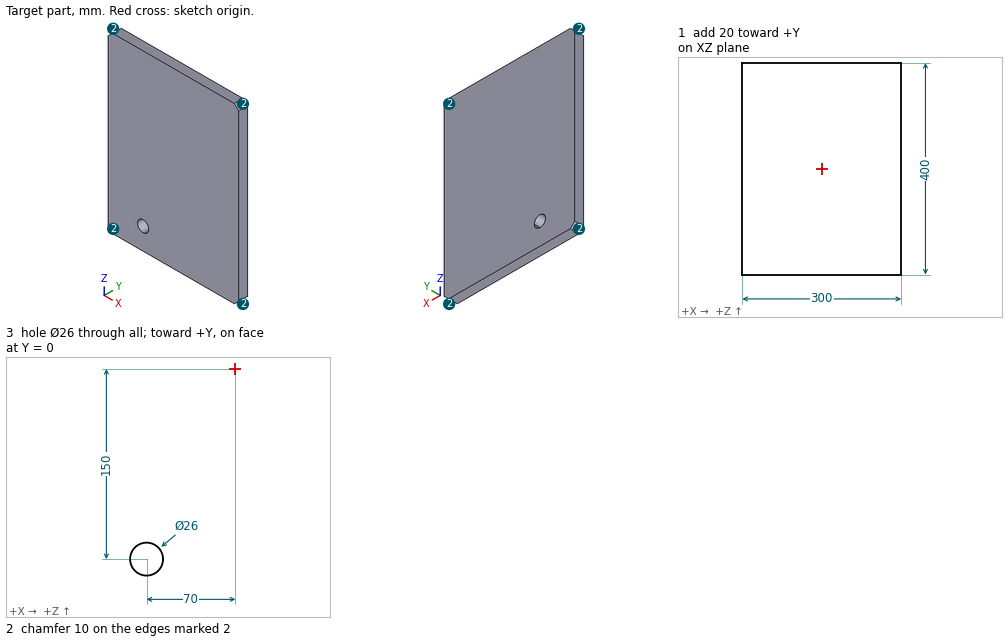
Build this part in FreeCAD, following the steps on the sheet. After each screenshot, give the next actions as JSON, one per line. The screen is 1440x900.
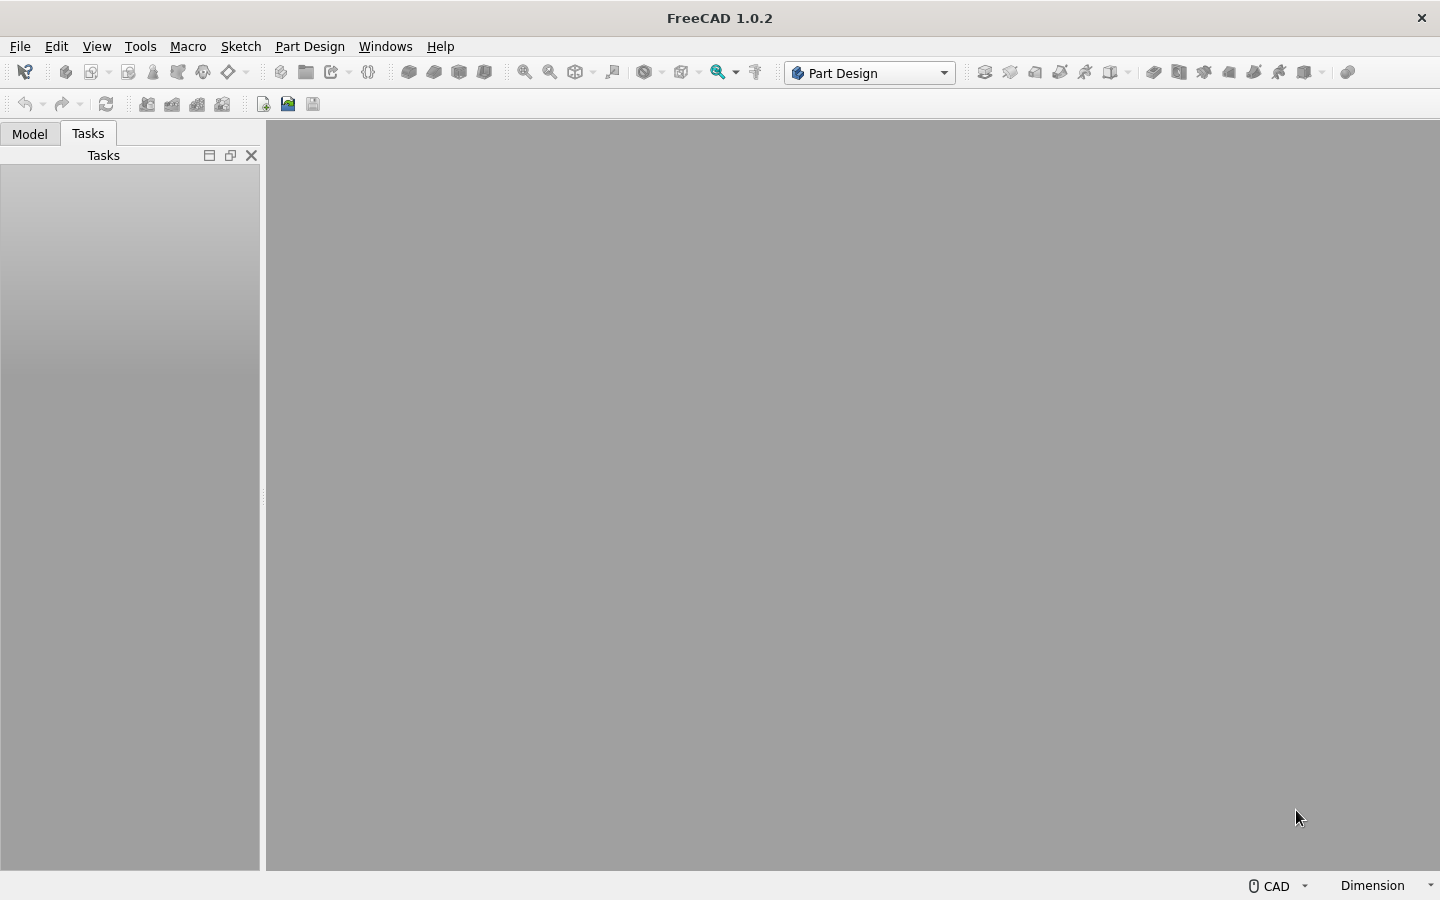
{"action": "left_click", "coordinate": [263, 104]}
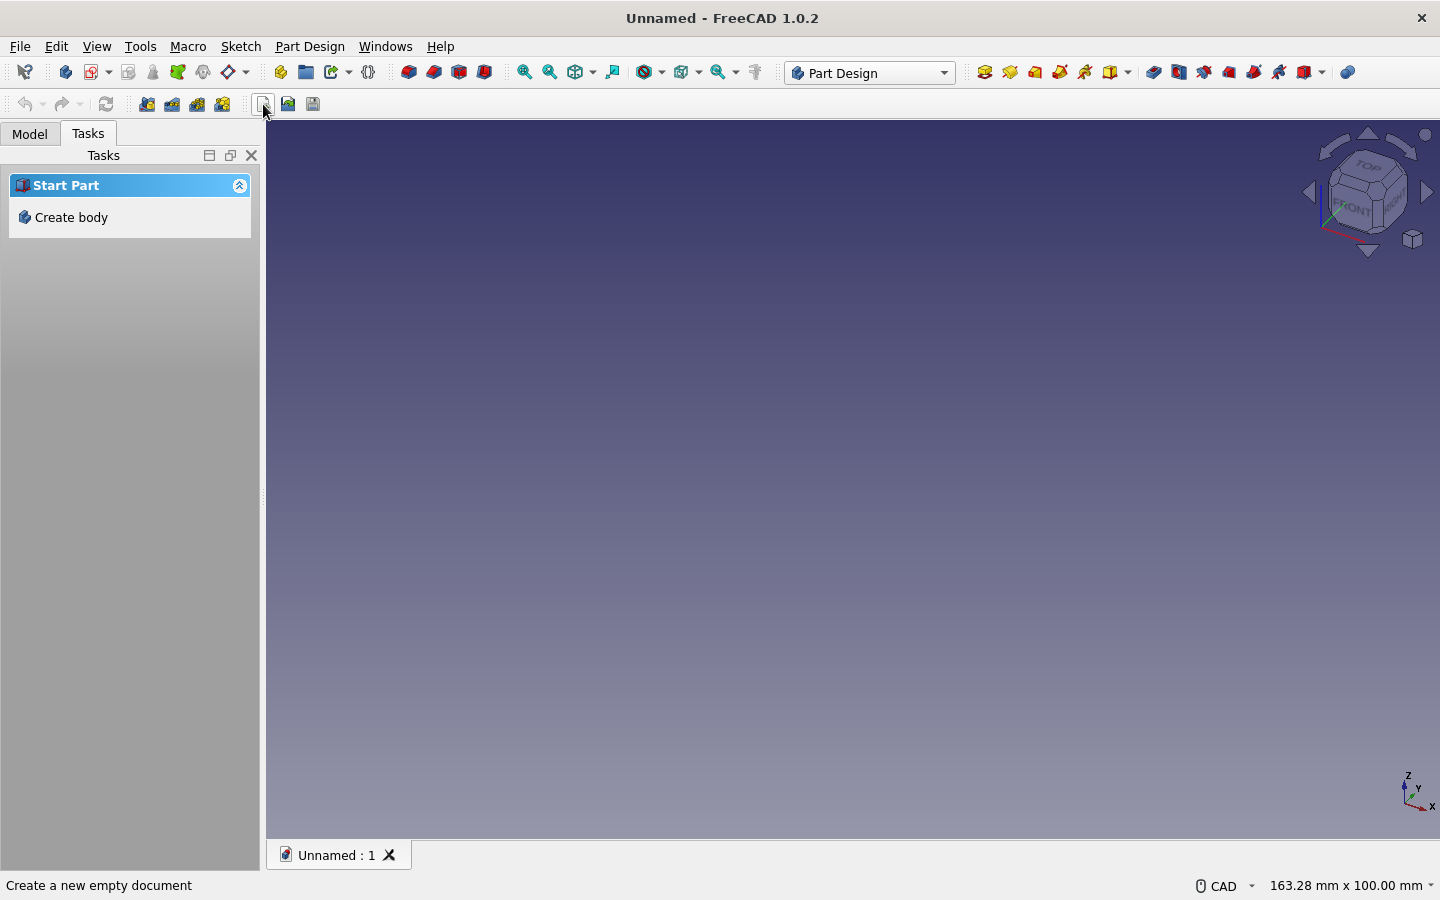
{"action": "left_click", "coordinate": [90, 72]}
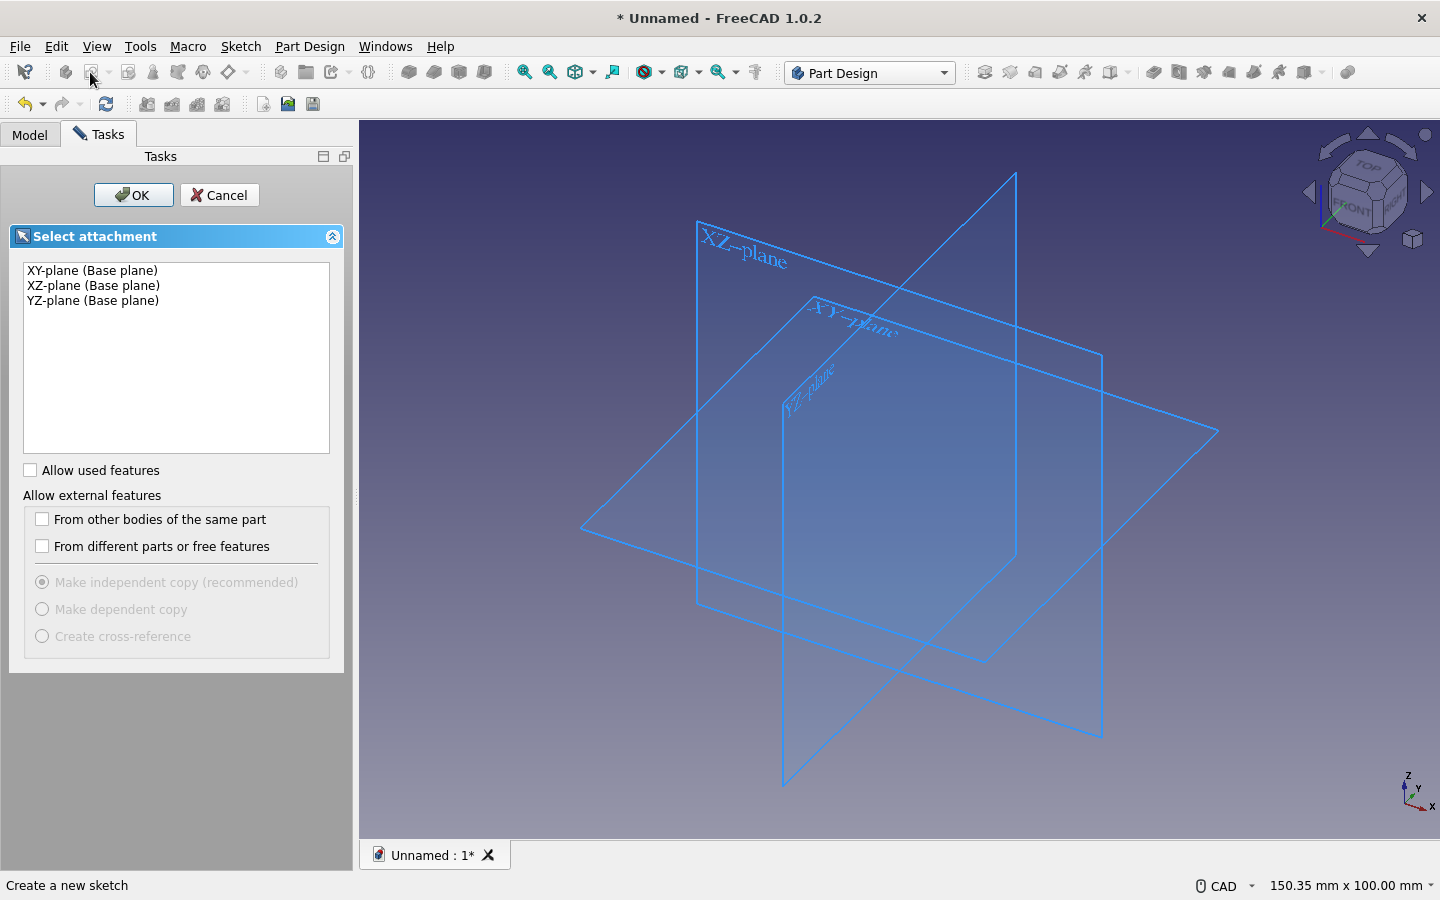
{"action": "left_click", "coordinate": [84, 286]}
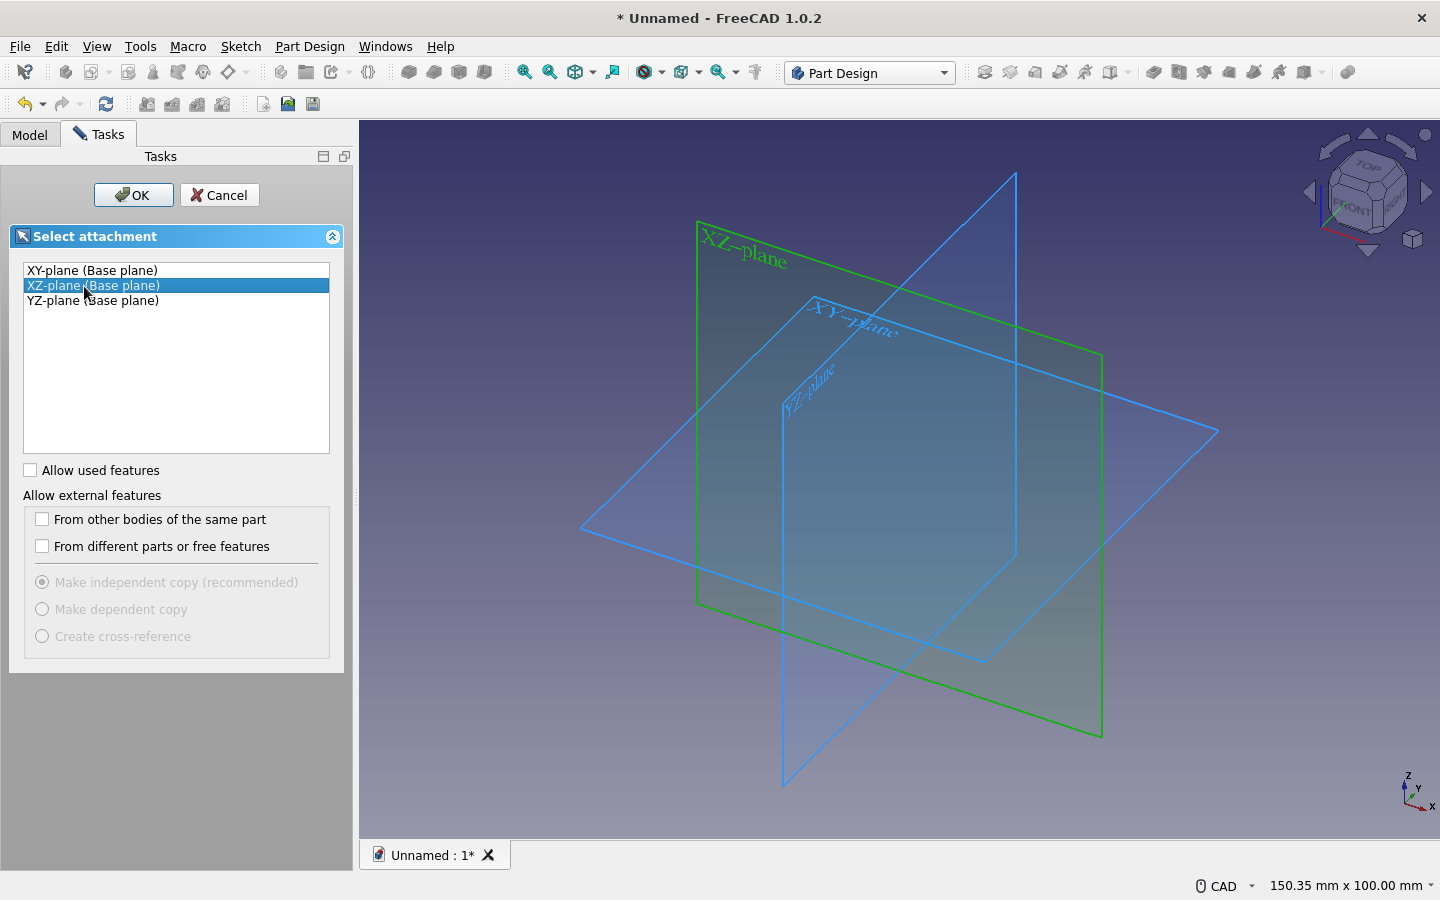
{"action": "left_click", "coordinate": [134, 195]}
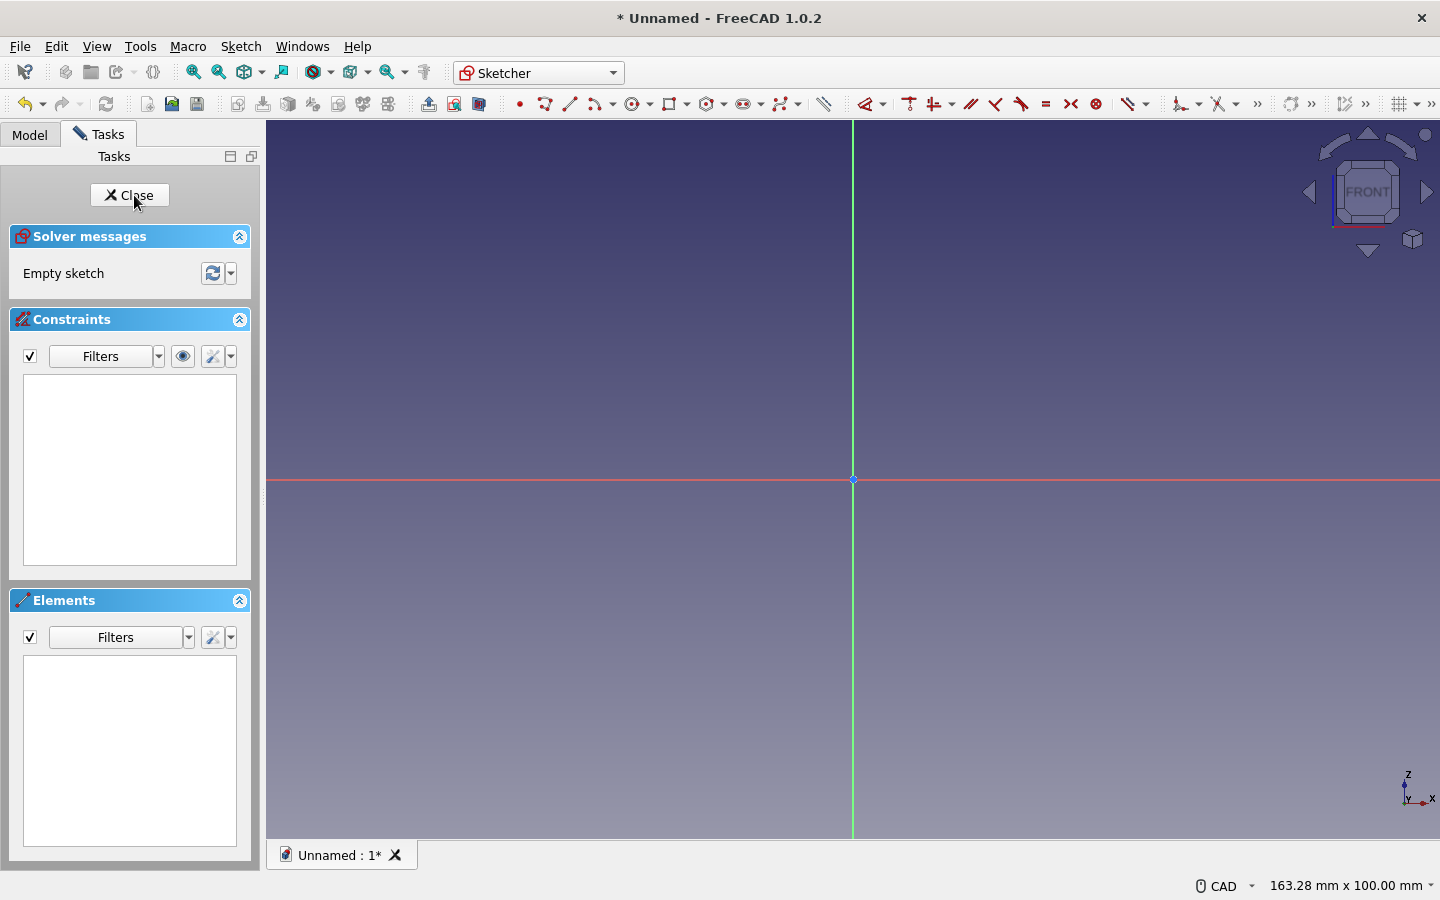
{"action": "scroll", "coordinate": [771, 480], "scroll_direction": "down", "scroll_amount": 9}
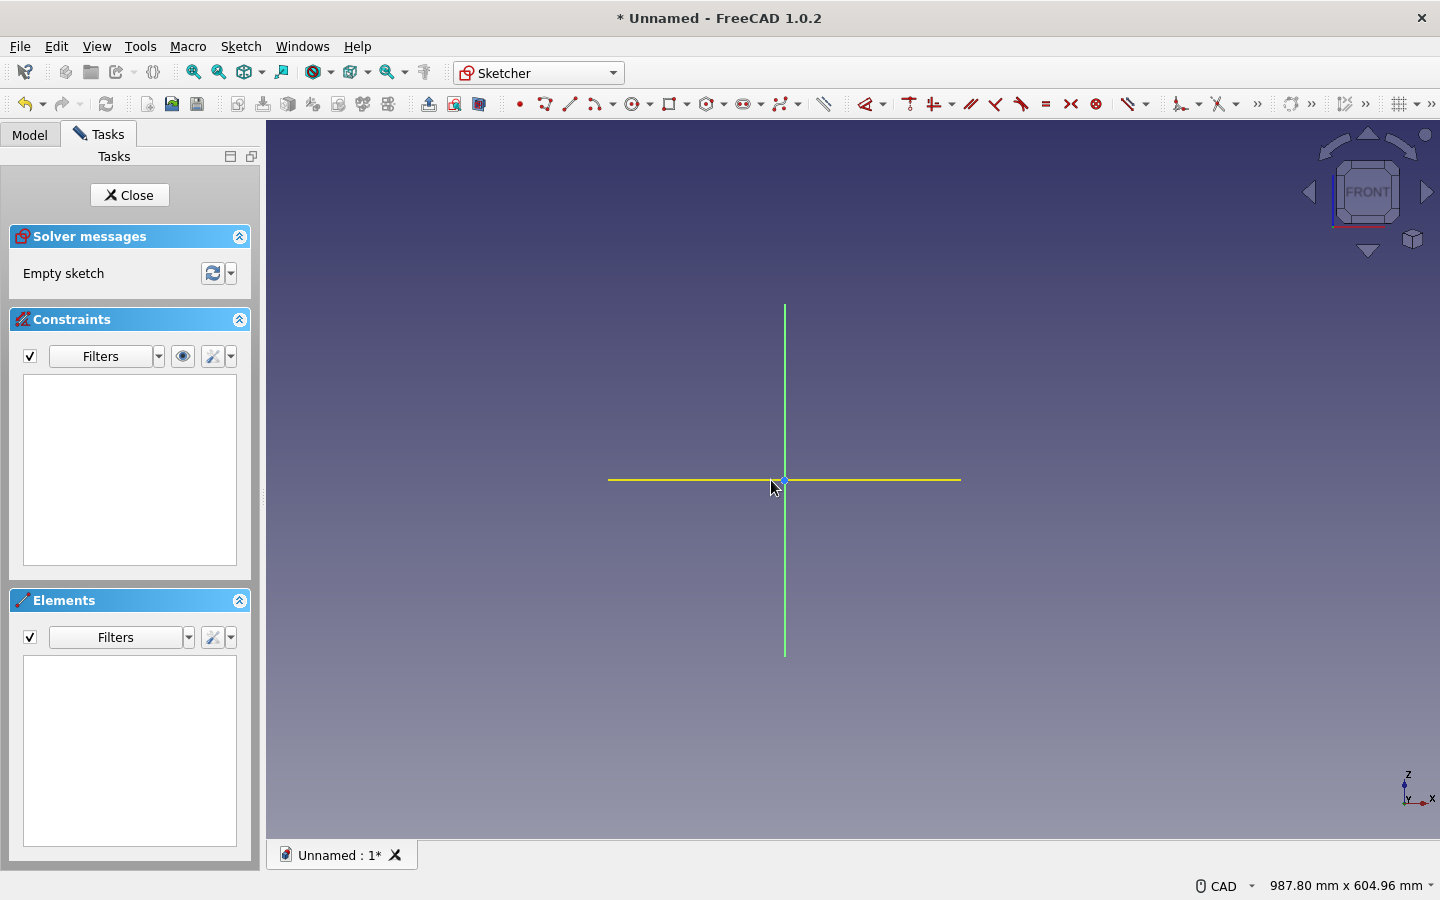
{"action": "left_click", "coordinate": [686, 104]}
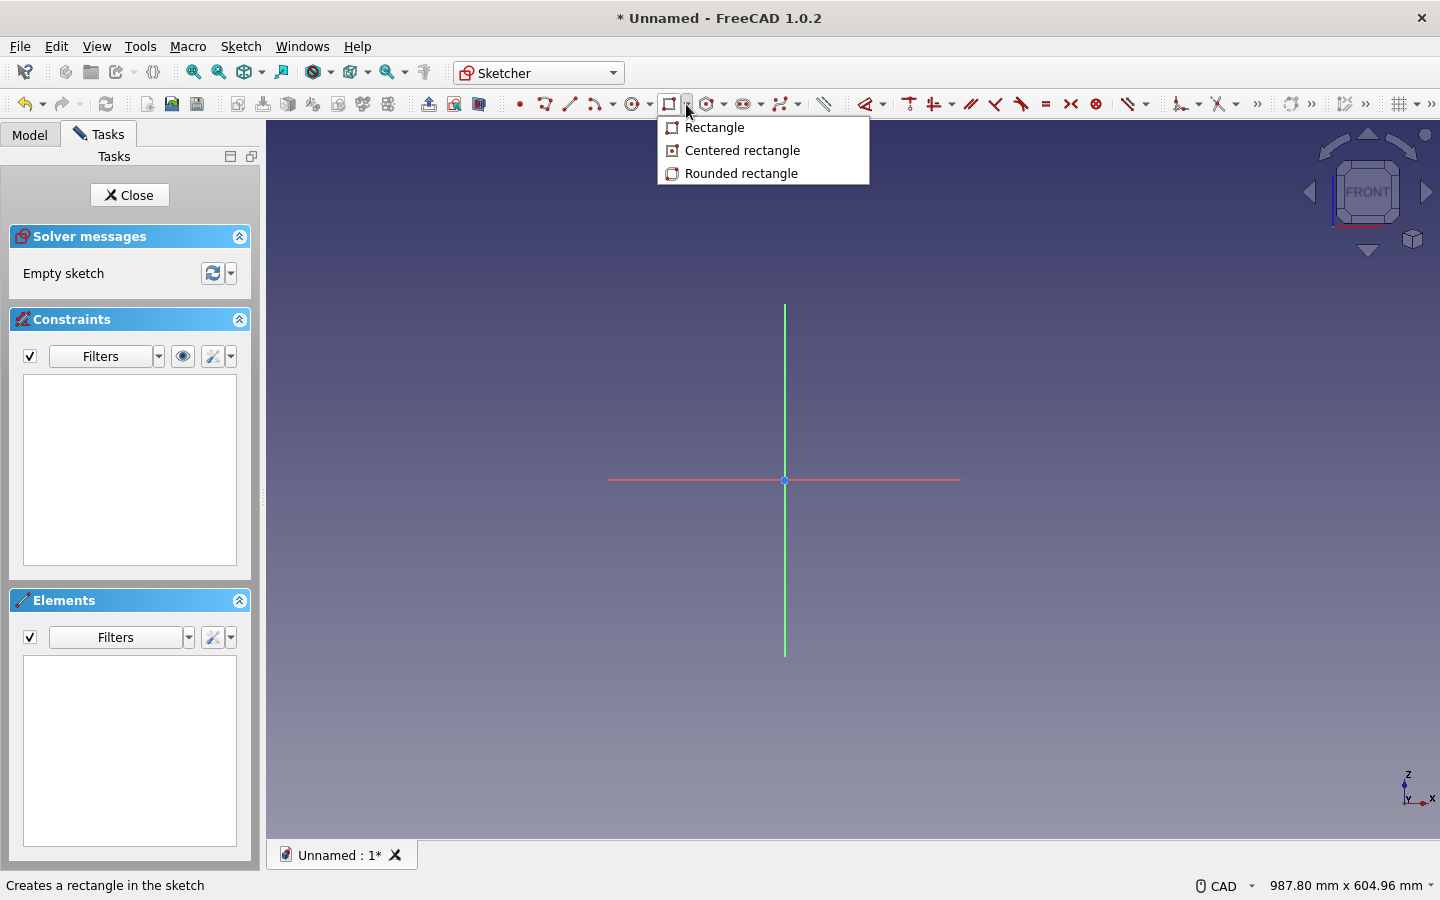
{"action": "left_click", "coordinate": [764, 150]}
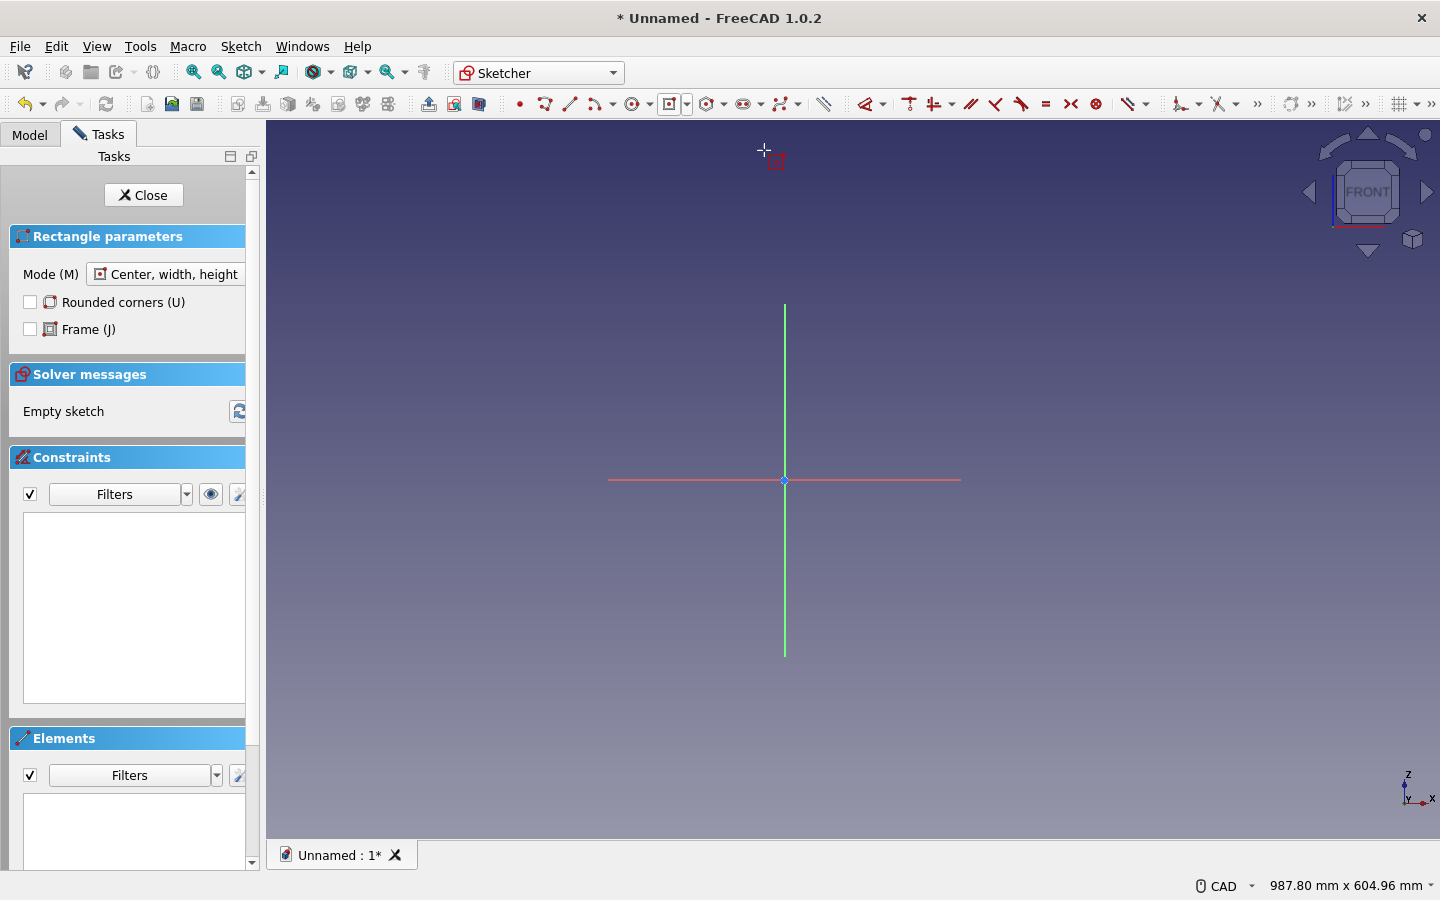
{"action": "left_click", "coordinate": [785, 480]}
{"action": "left_click", "coordinate": [963, 243]}
{"action": "key", "text": "Escape"}